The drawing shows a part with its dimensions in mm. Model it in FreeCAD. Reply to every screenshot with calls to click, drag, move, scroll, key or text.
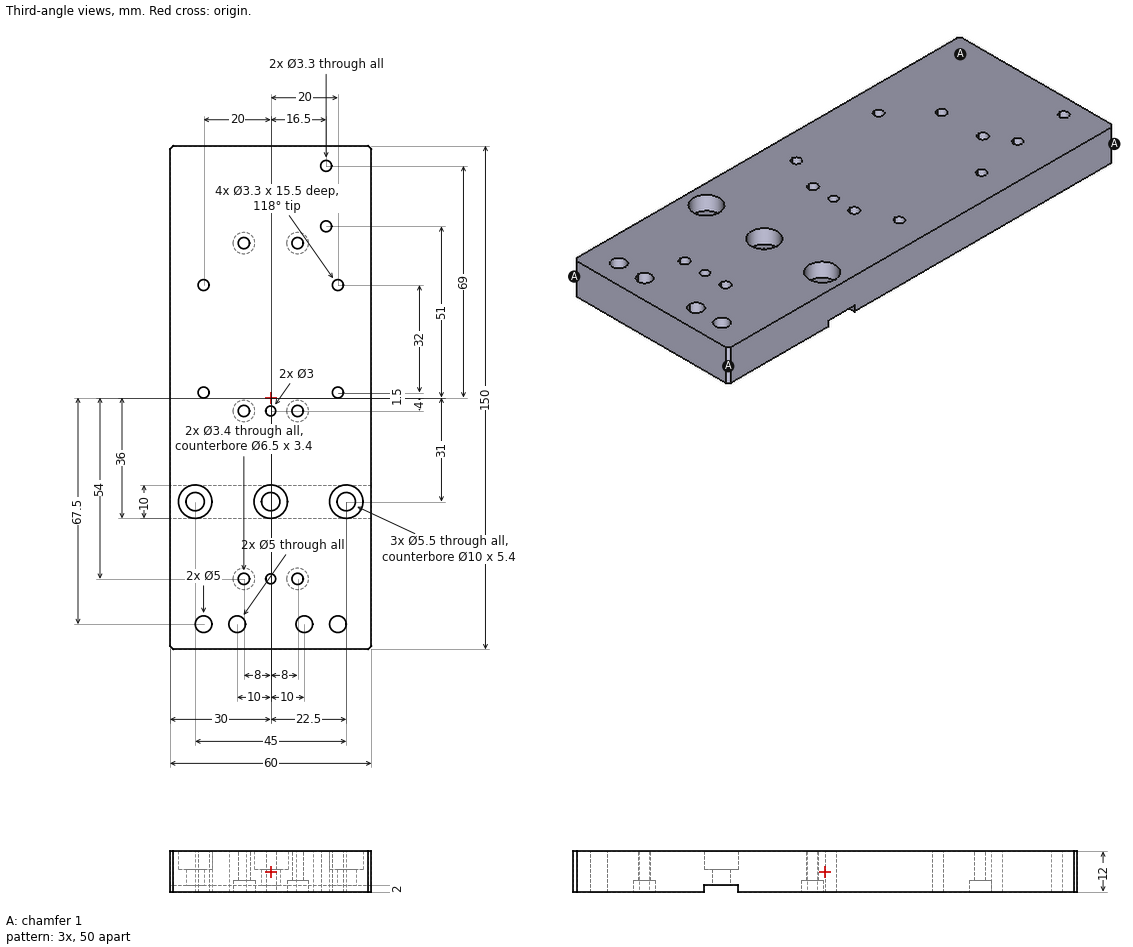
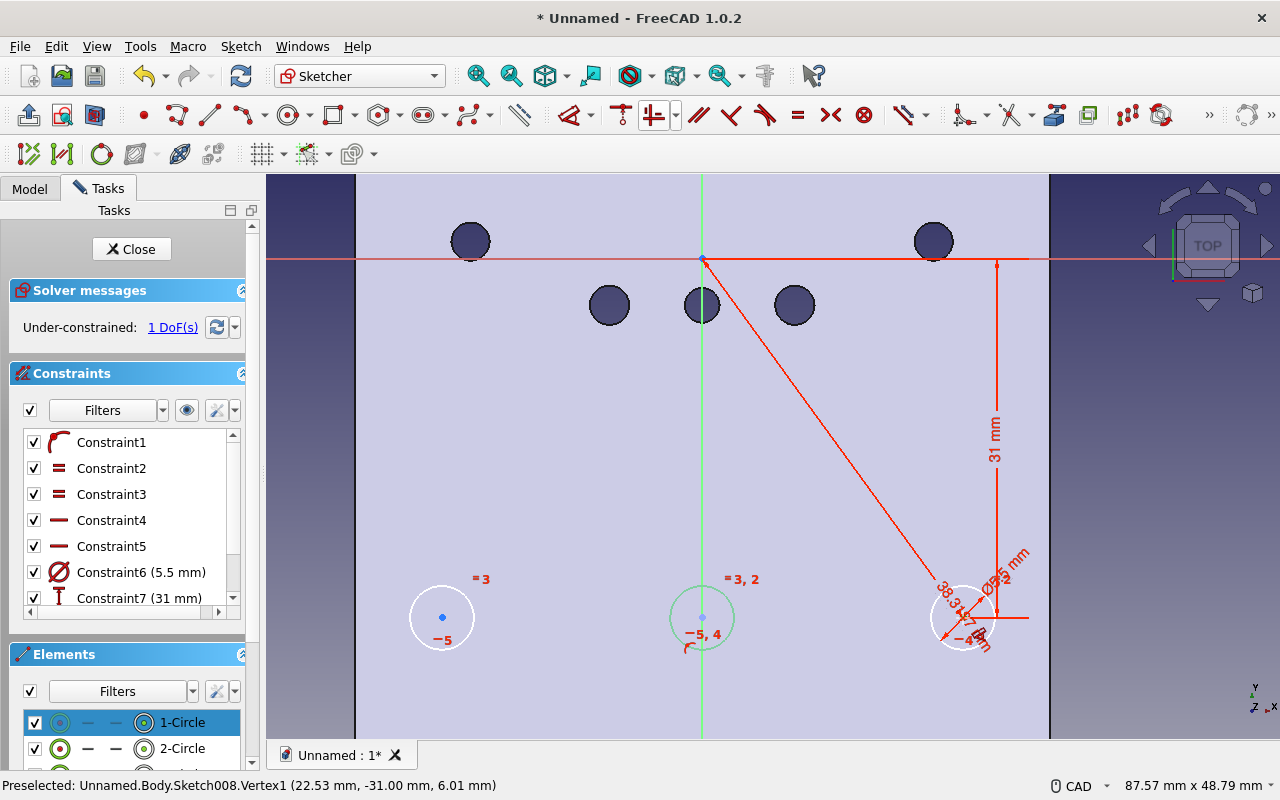
click(442, 618)
click(583, 652)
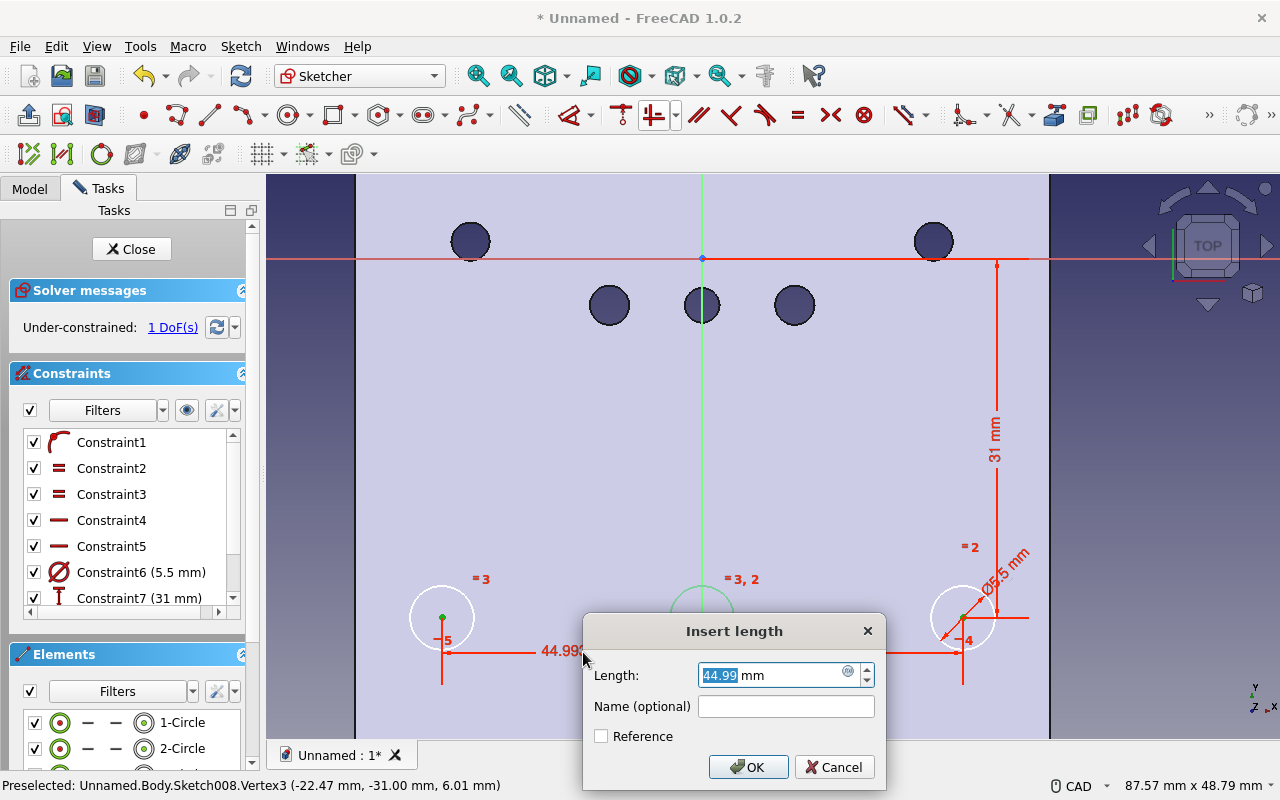
text(45)
key(Return)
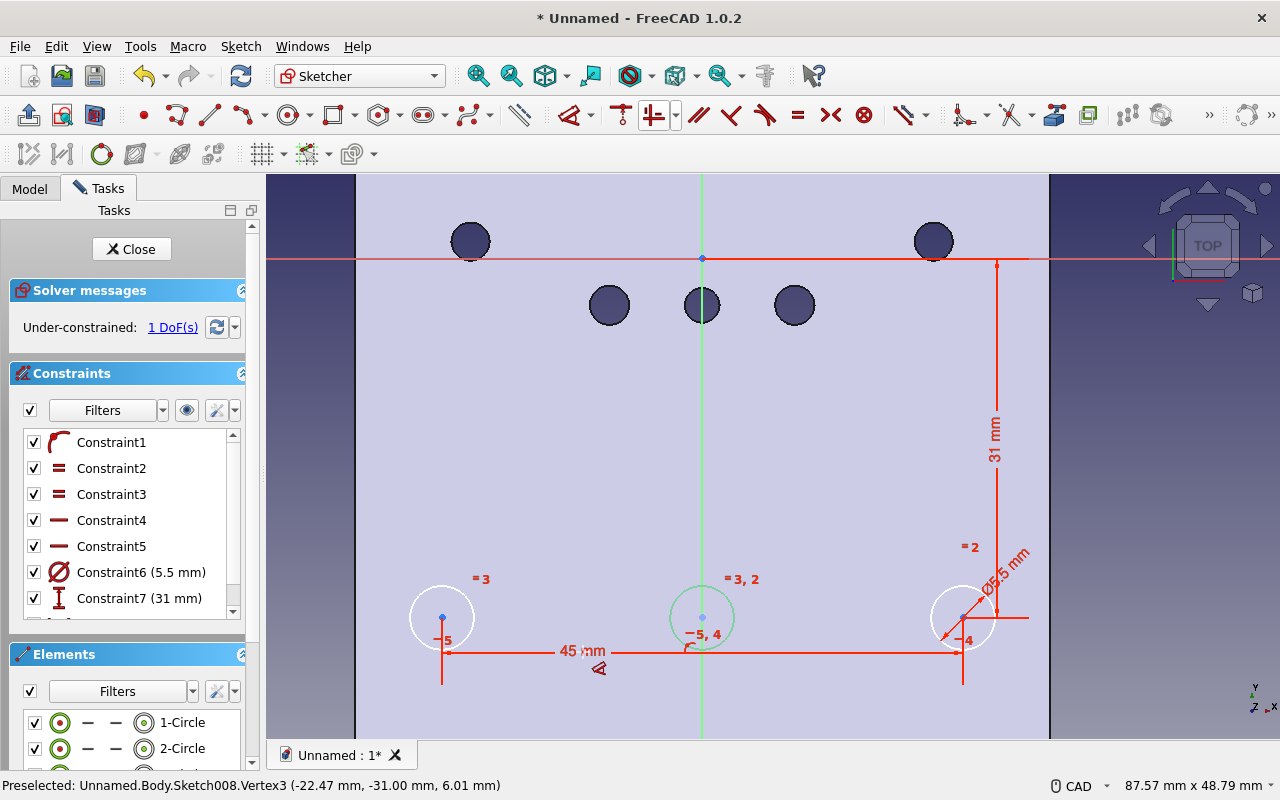
click(963, 618)
click(833, 225)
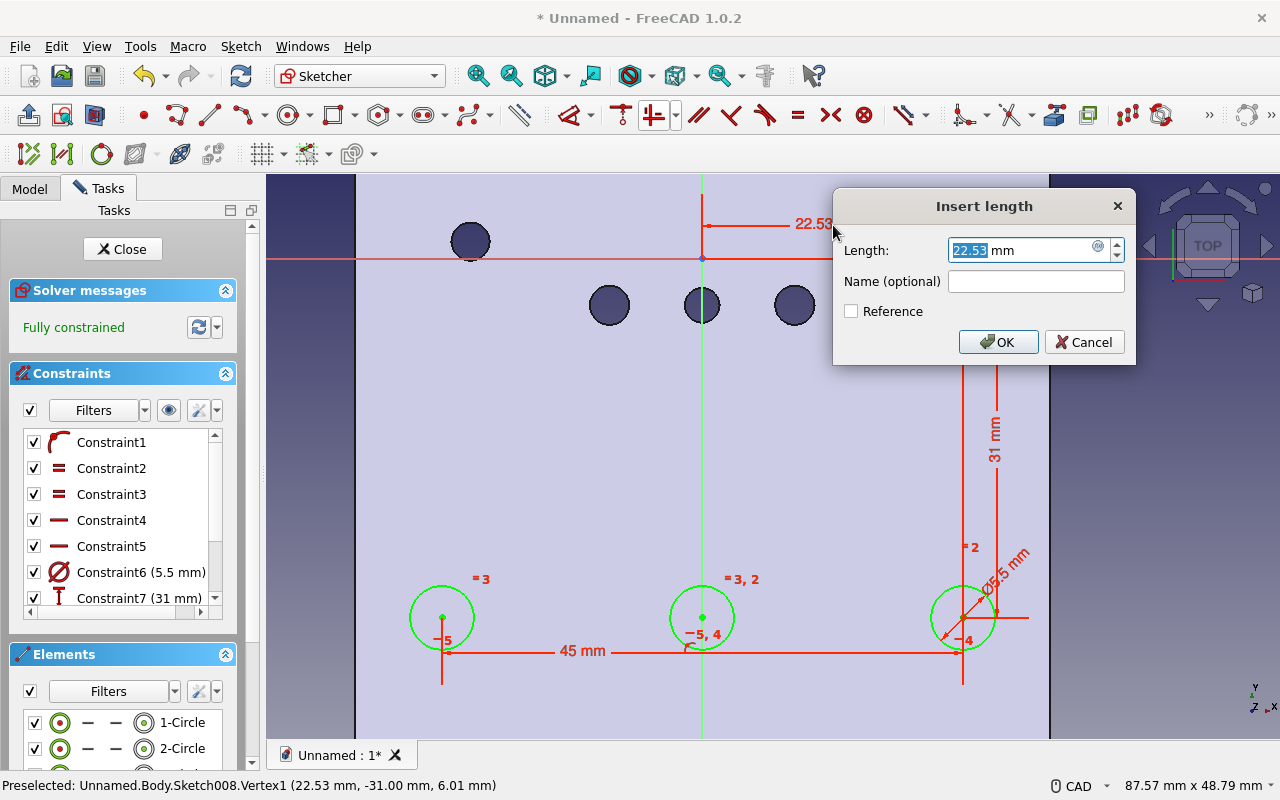
text(22.5)
key(Return)
key(Escape)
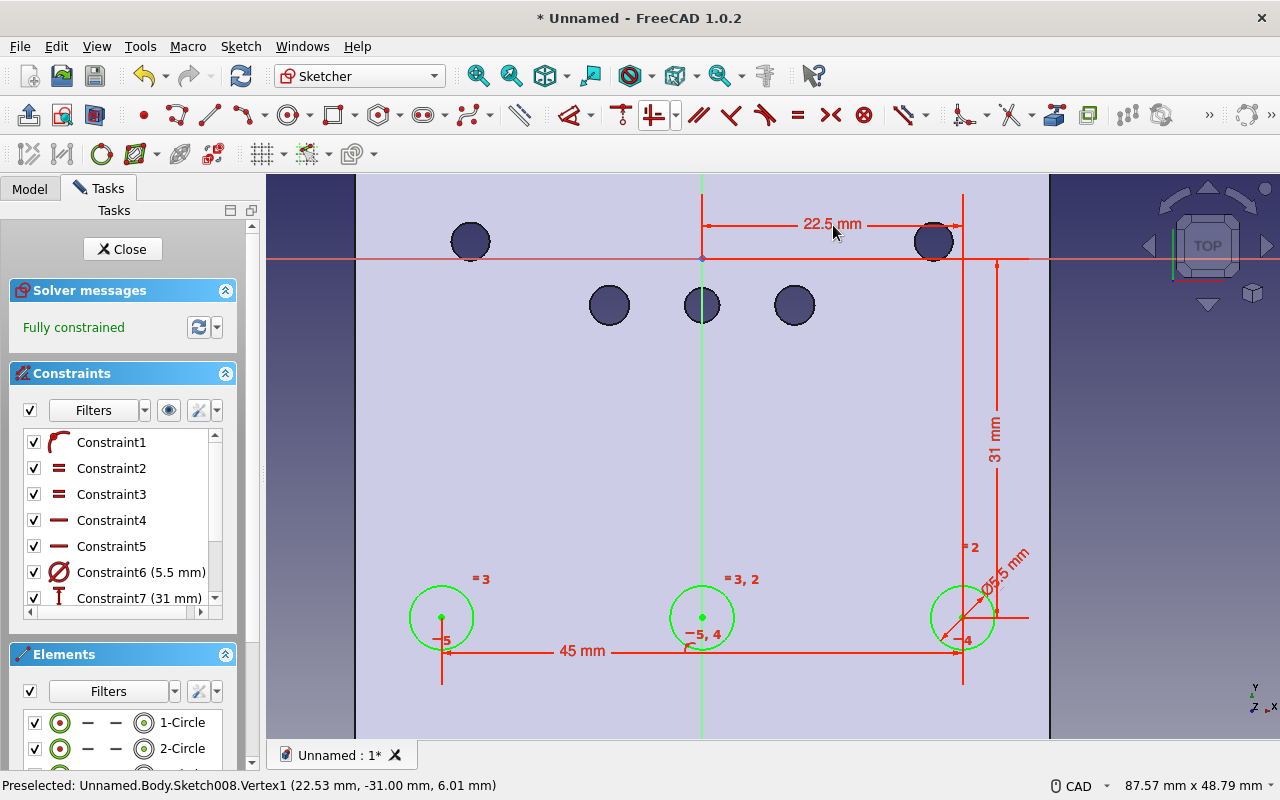
click(123, 249)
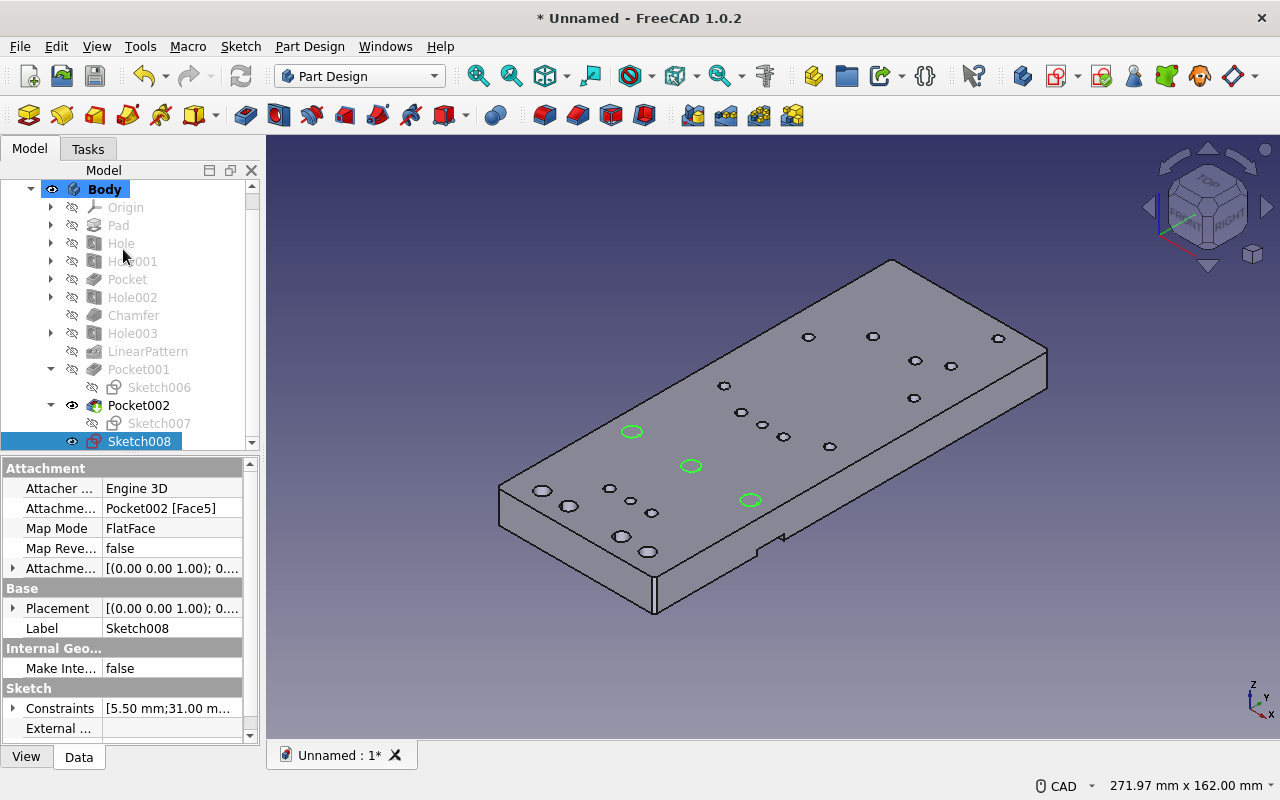
click(279, 116)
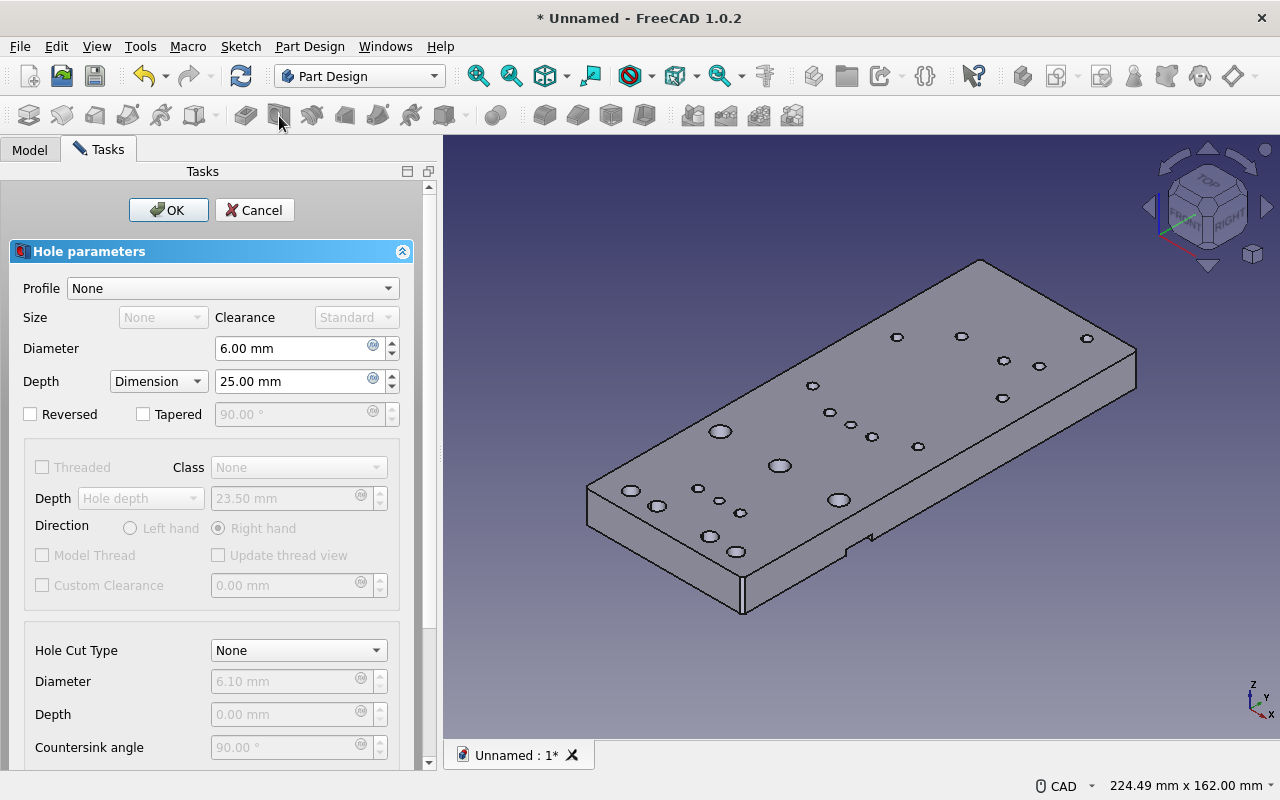
triple_click(300, 348)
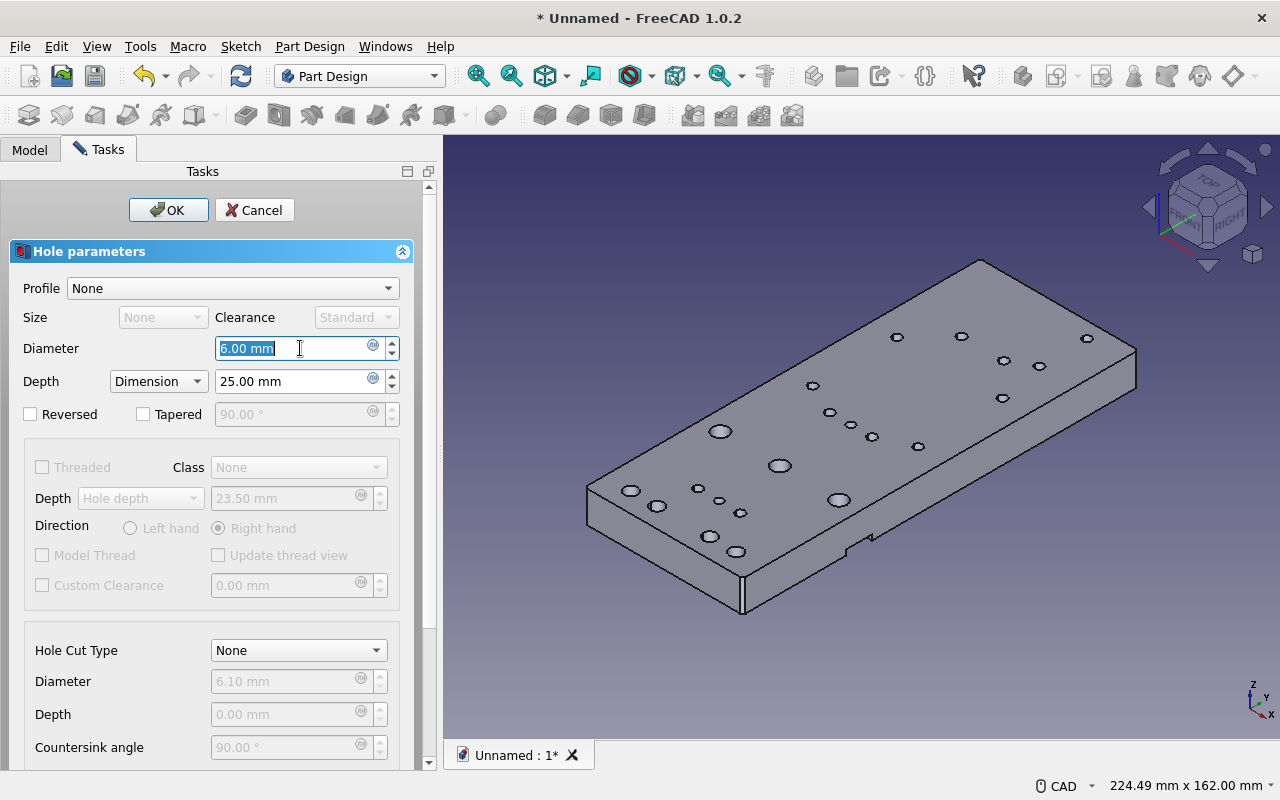
text(5.5)
key(Tab)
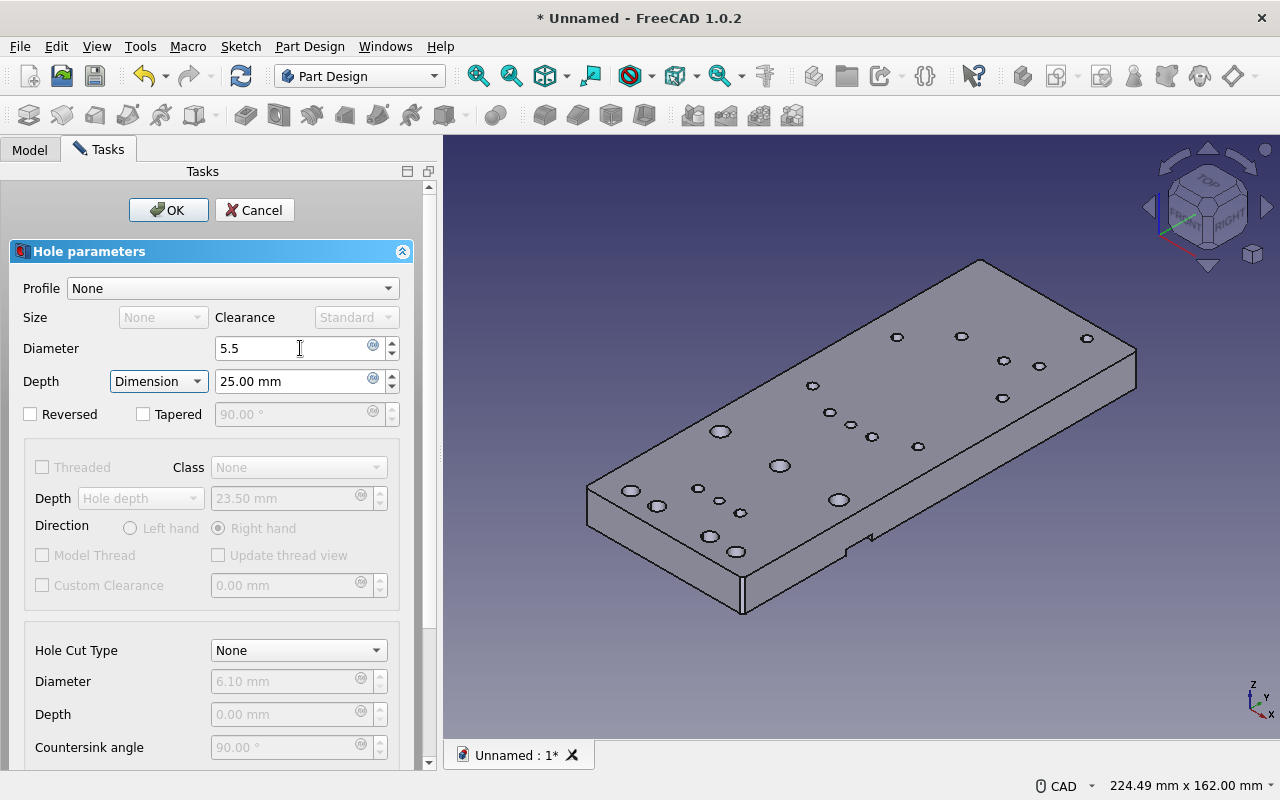
click(160, 382)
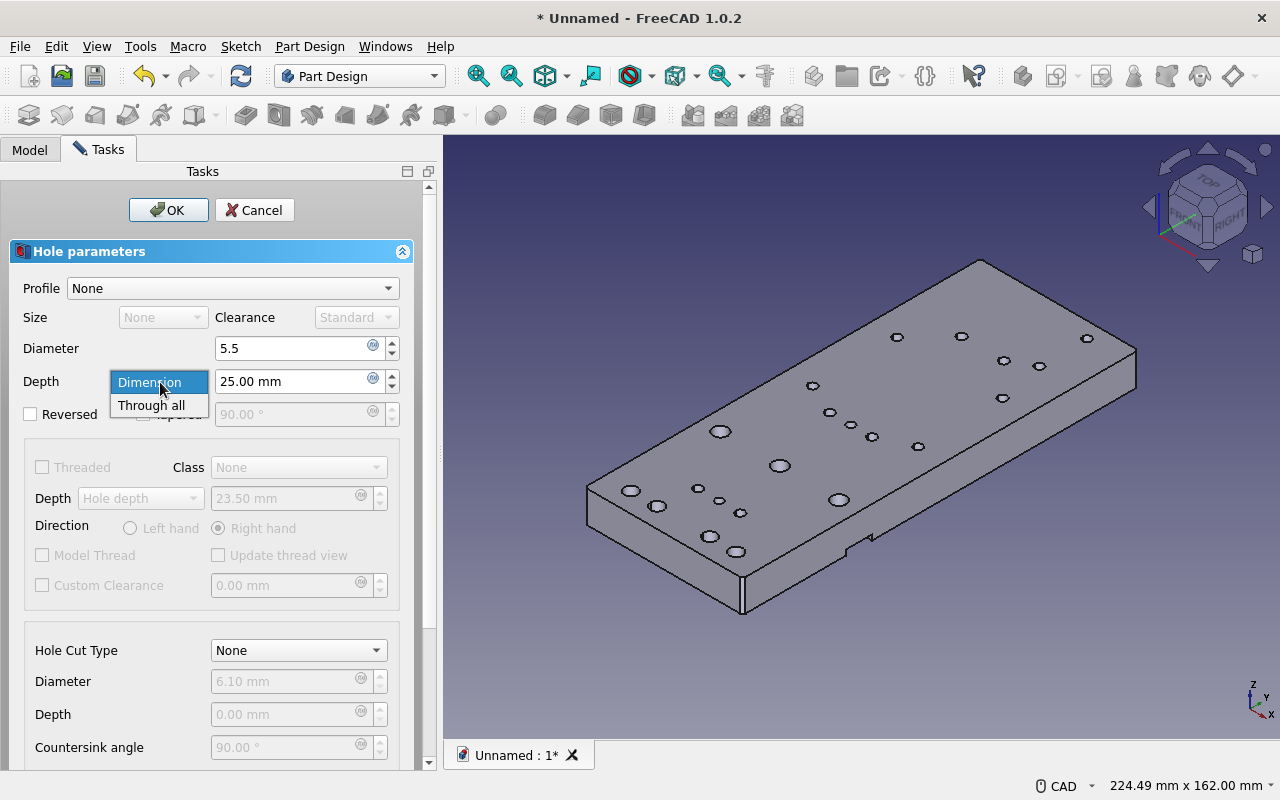
click(158, 406)